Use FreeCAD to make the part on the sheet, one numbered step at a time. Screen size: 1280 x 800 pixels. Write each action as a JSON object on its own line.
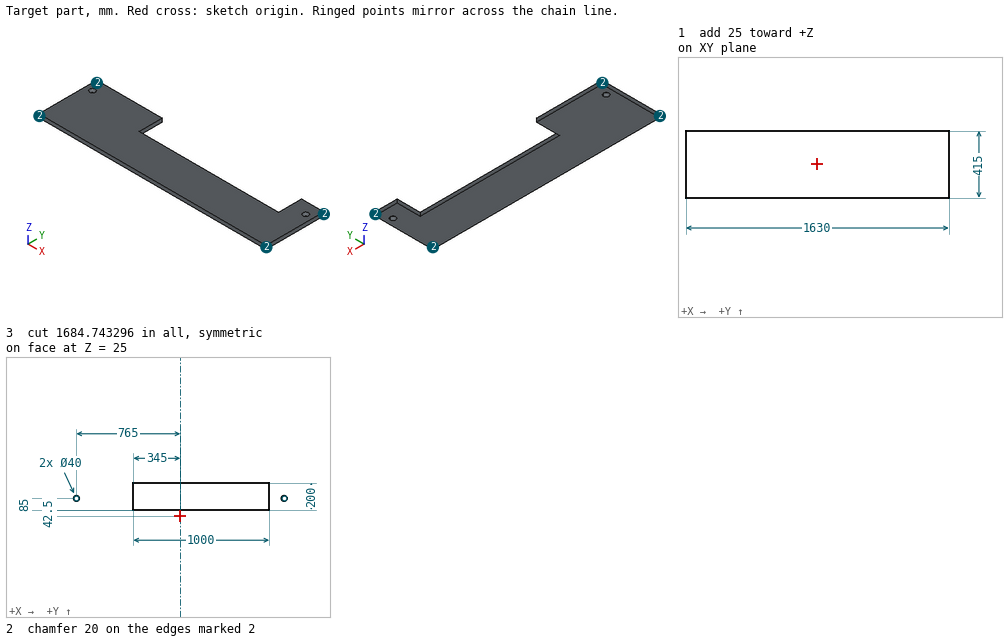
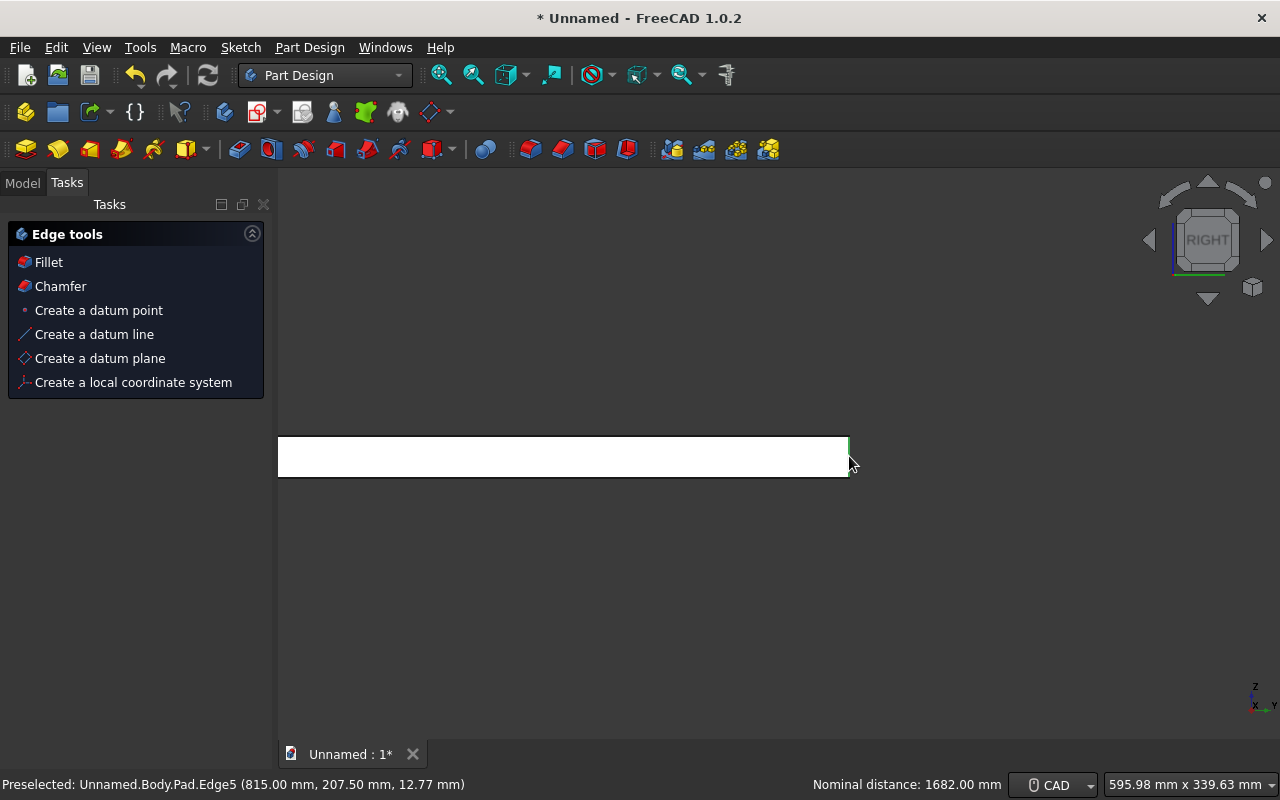
{"action": "left_click", "coordinate": [442, 76]}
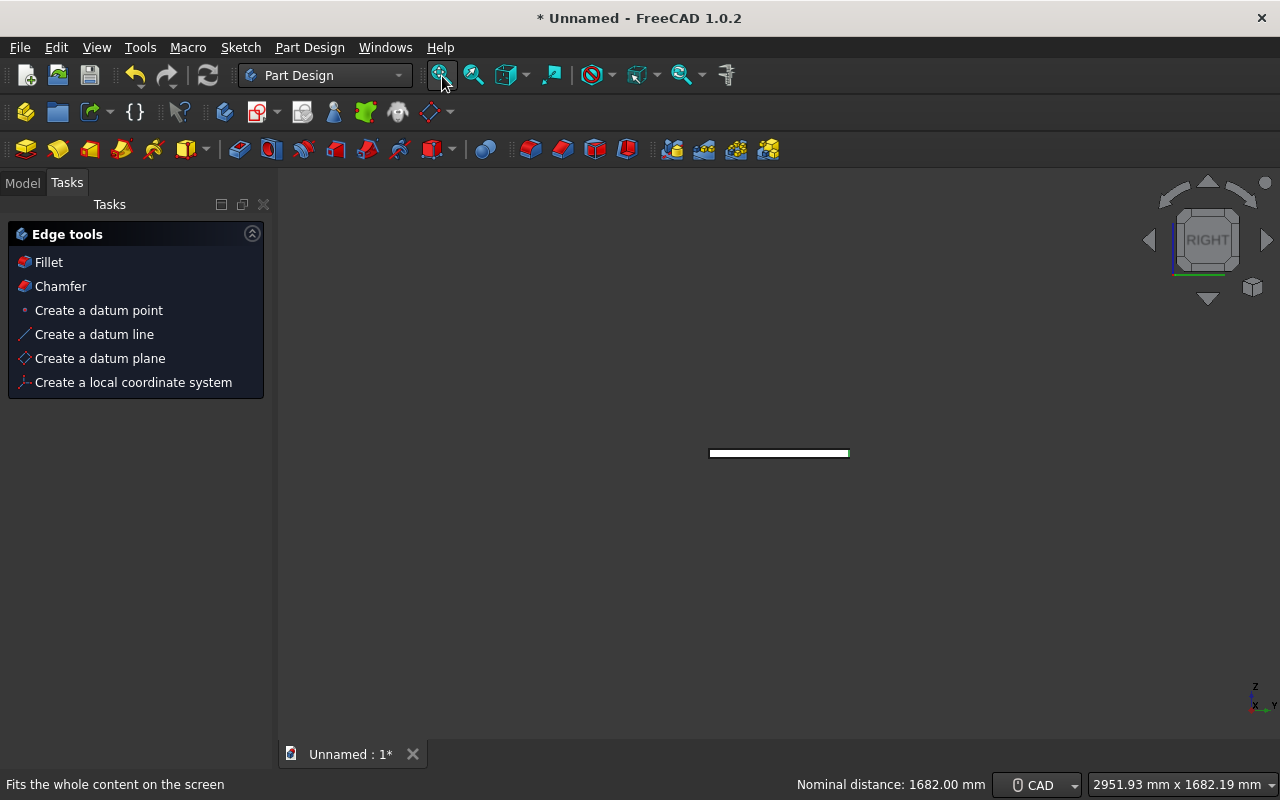
{"action": "key", "text": "5"}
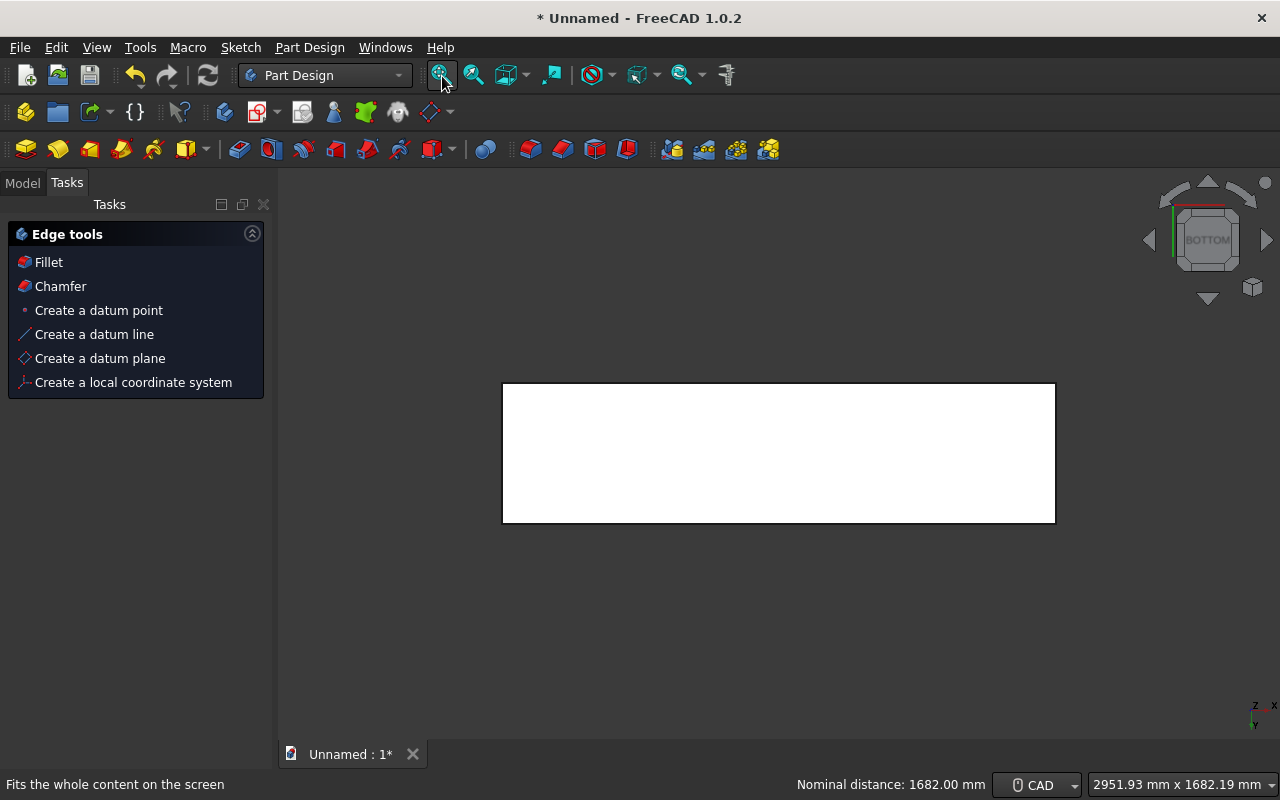
{"action": "scroll", "coordinate": [502, 523], "scroll_direction": "up", "scroll_amount": 8}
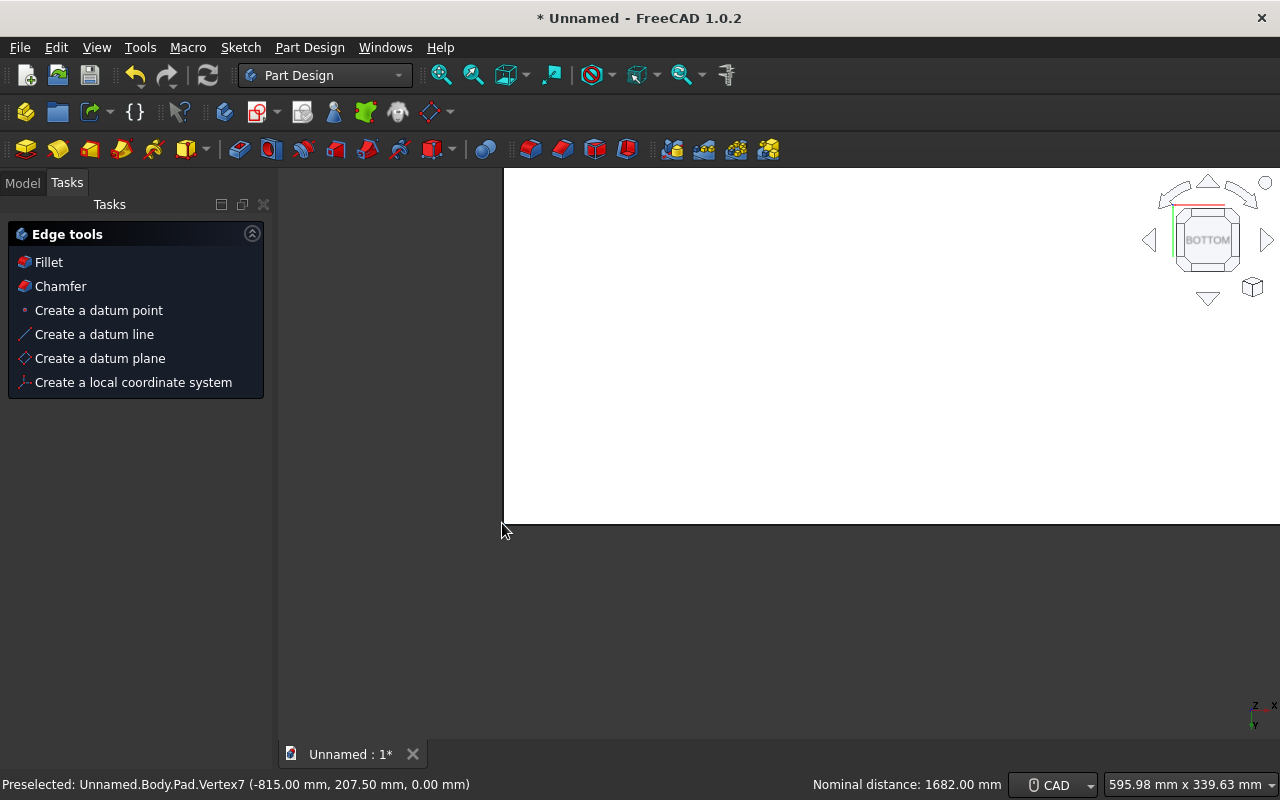
{"action": "left_click", "coordinate": [442, 76]}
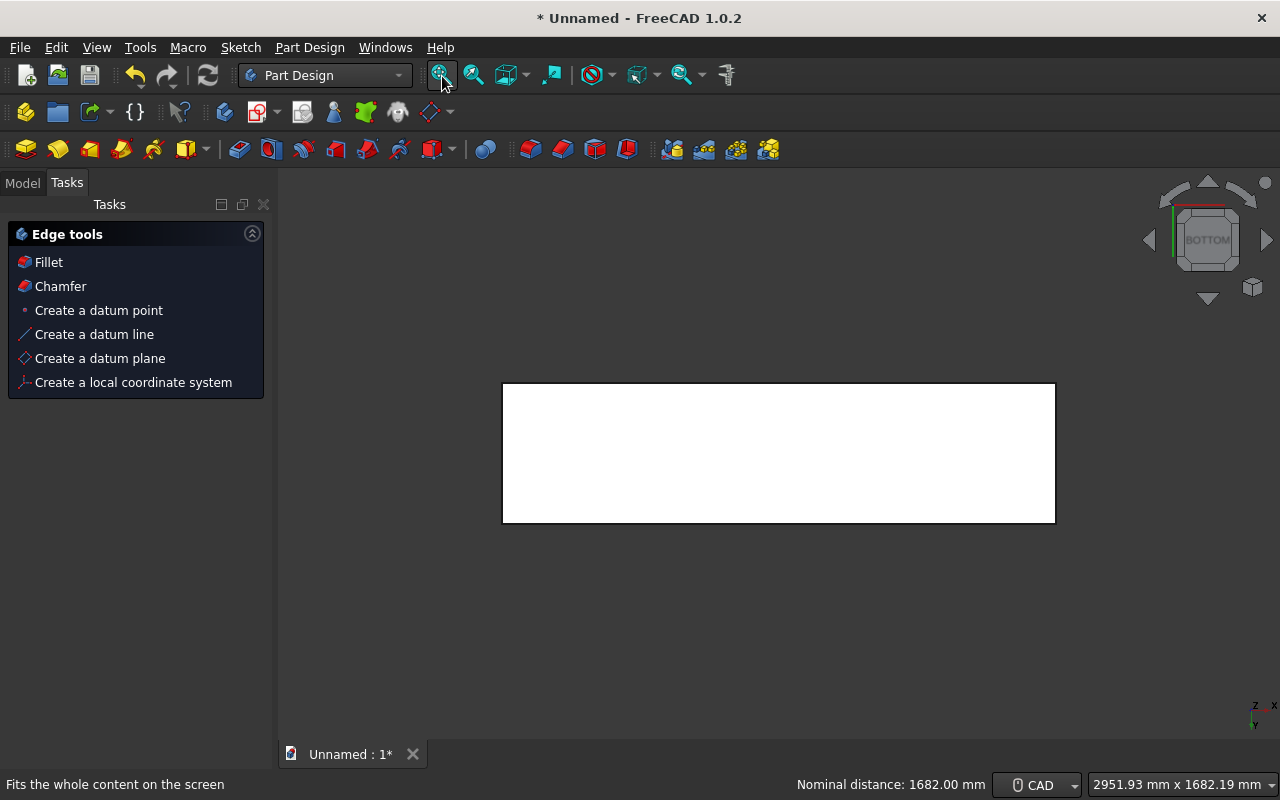
{"action": "key", "text": "4"}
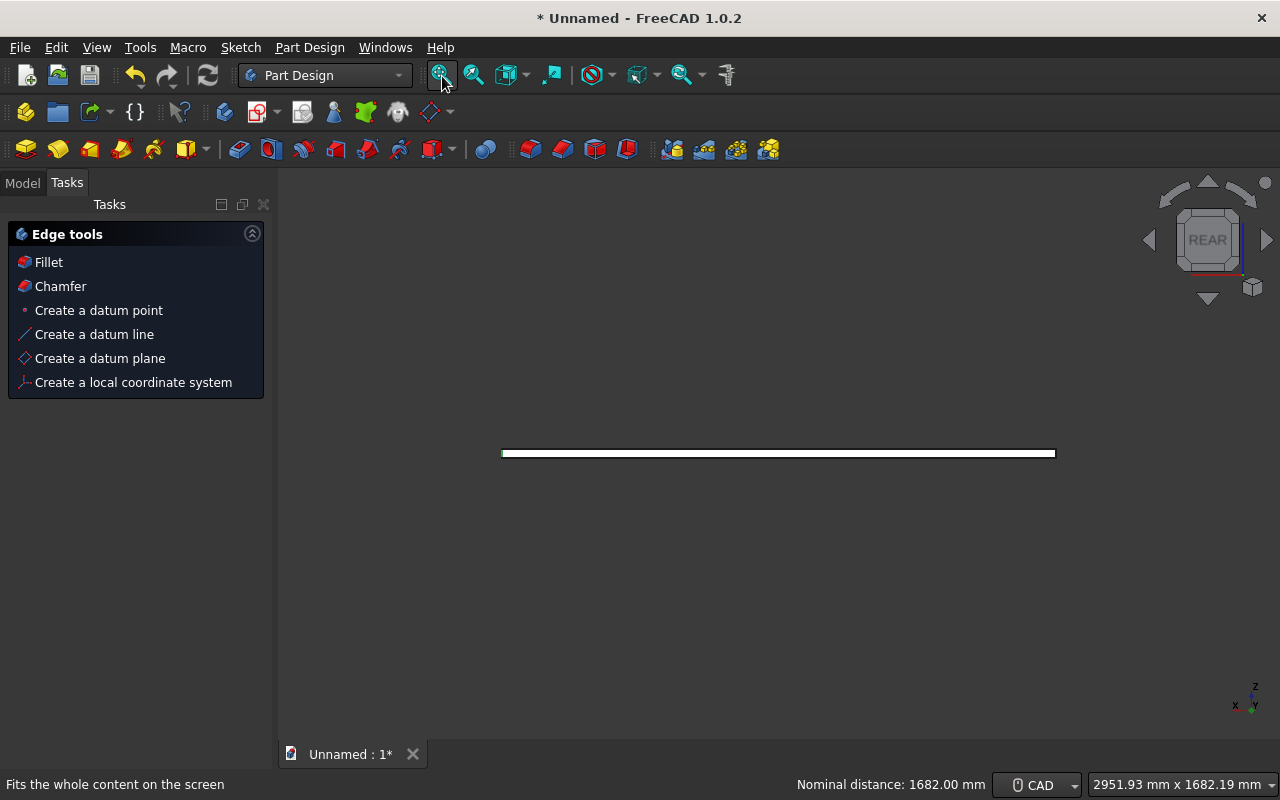
{"action": "scroll", "coordinate": [1056, 453], "scroll_direction": "up", "scroll_amount": 8}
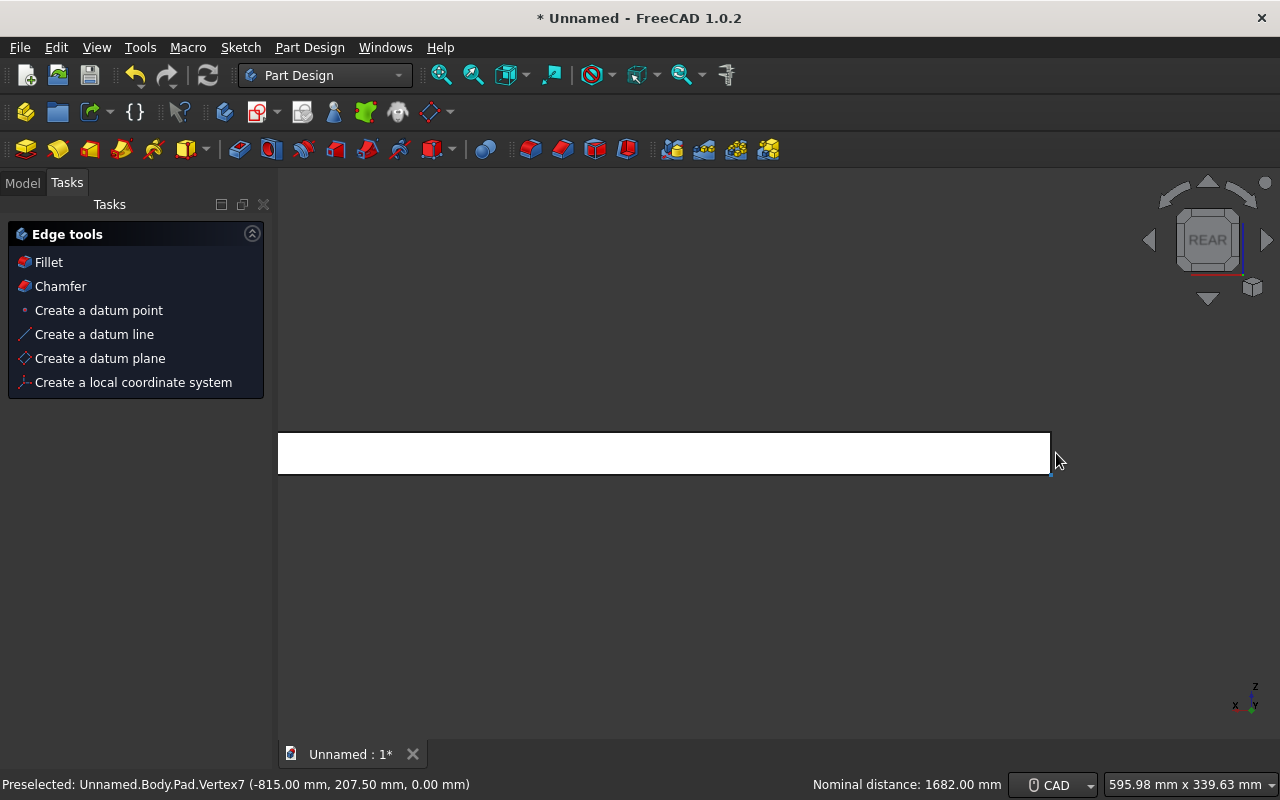
{"action": "left_click", "coordinate": [1051, 453], "text": "ctrl"}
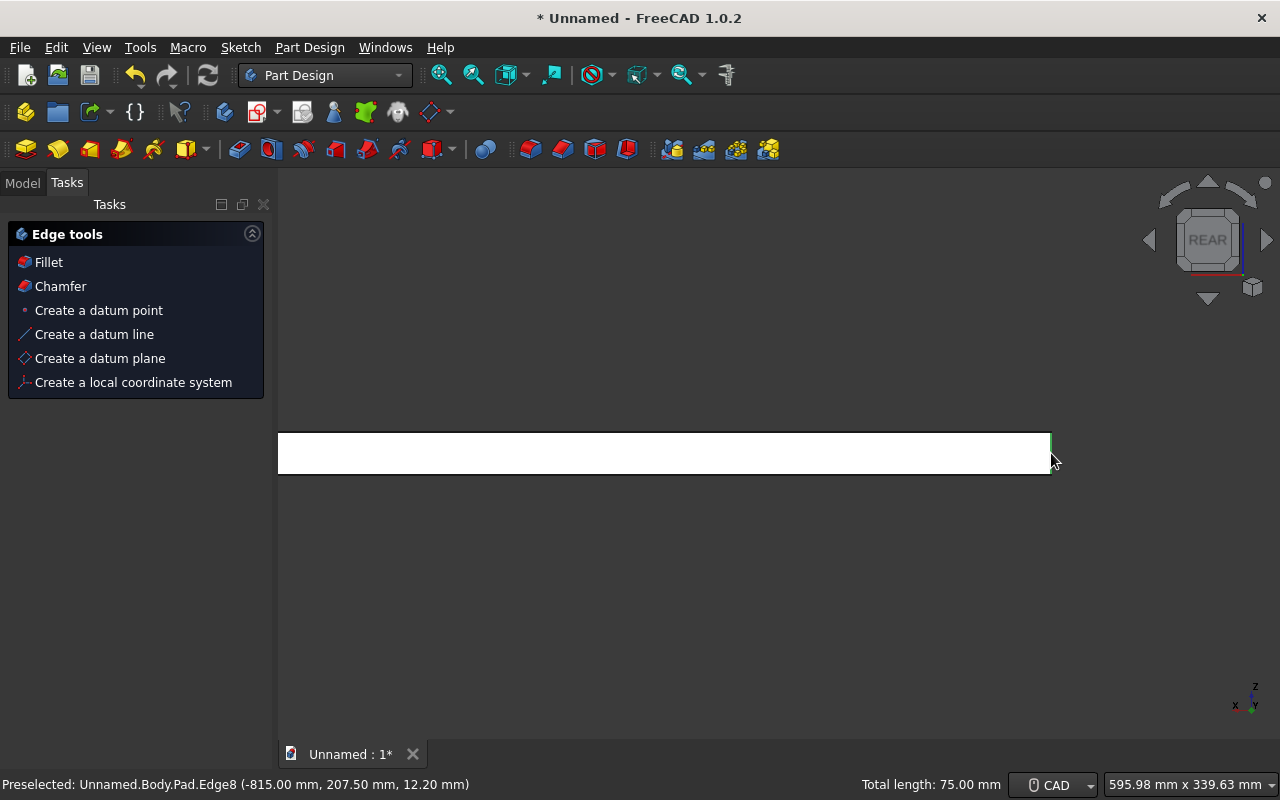
{"action": "key", "text": "v f"}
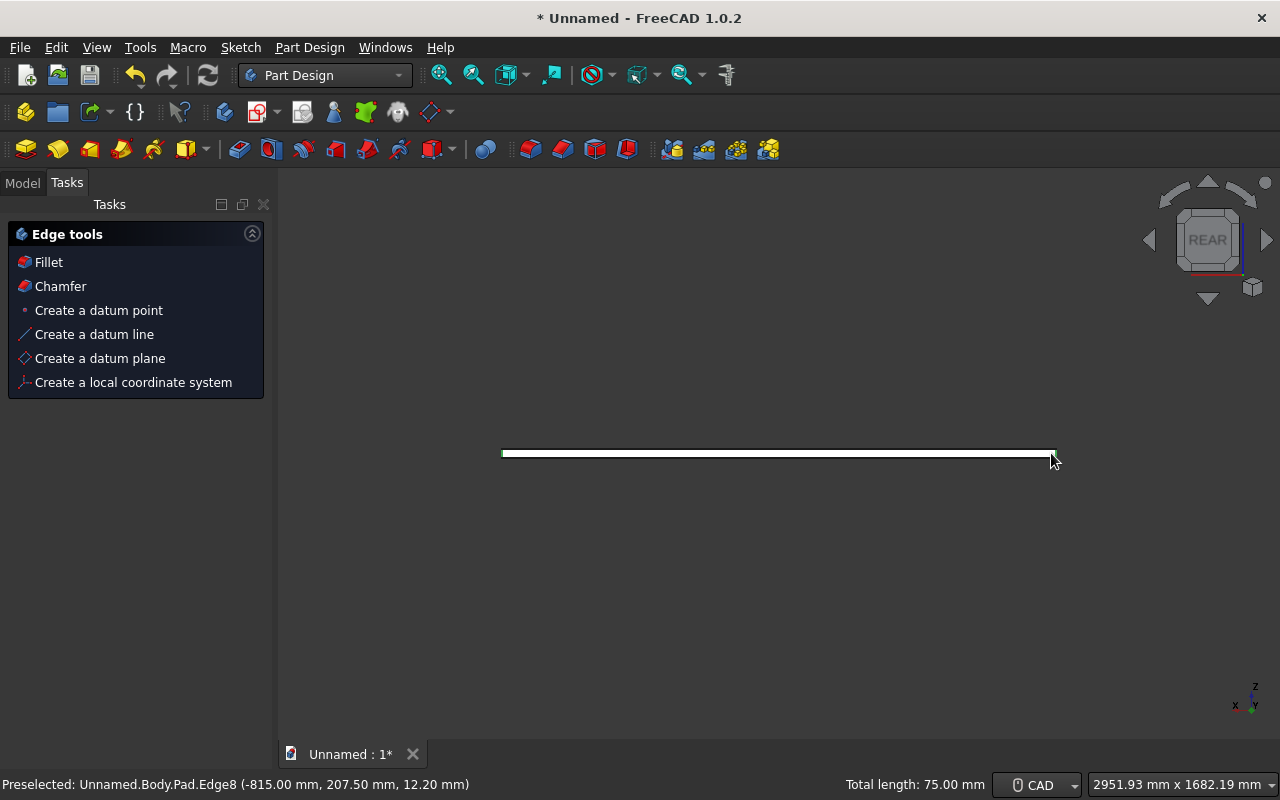
{"action": "key", "text": "6"}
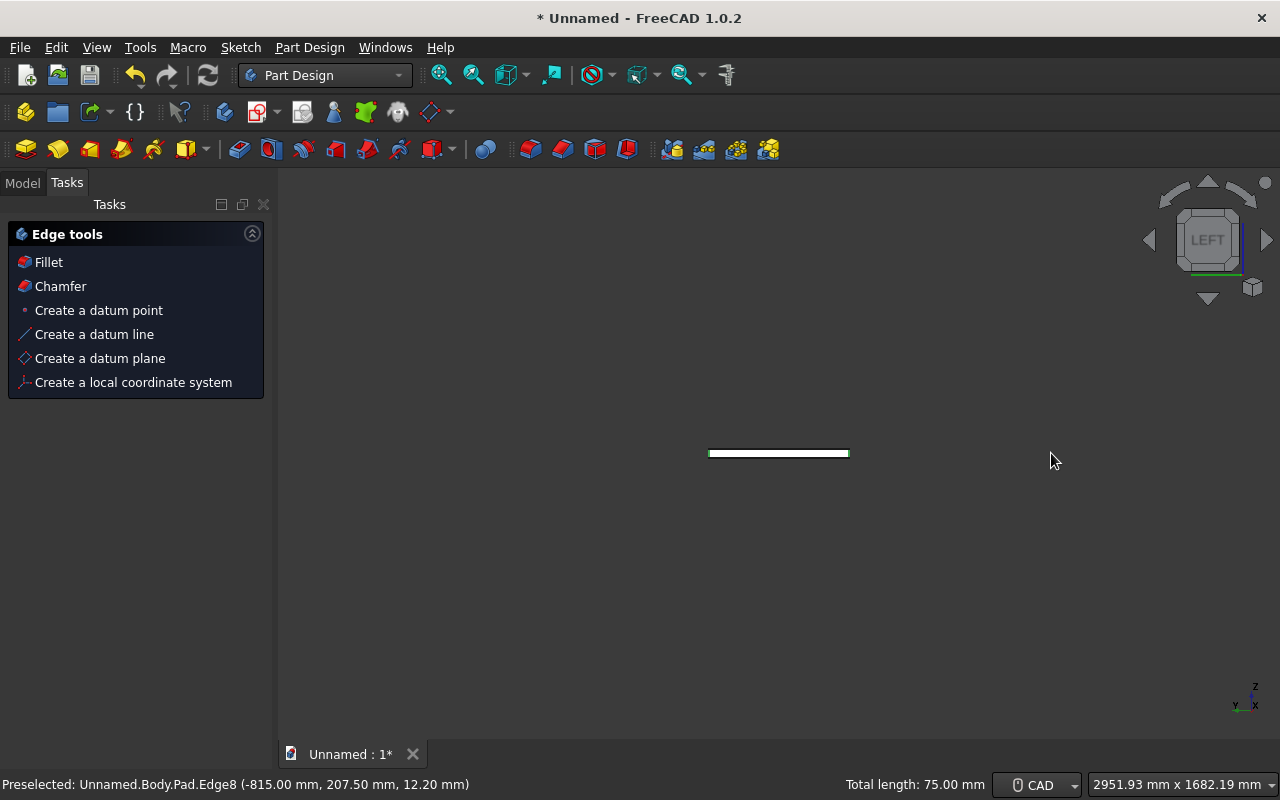
{"action": "left_click", "coordinate": [442, 76]}